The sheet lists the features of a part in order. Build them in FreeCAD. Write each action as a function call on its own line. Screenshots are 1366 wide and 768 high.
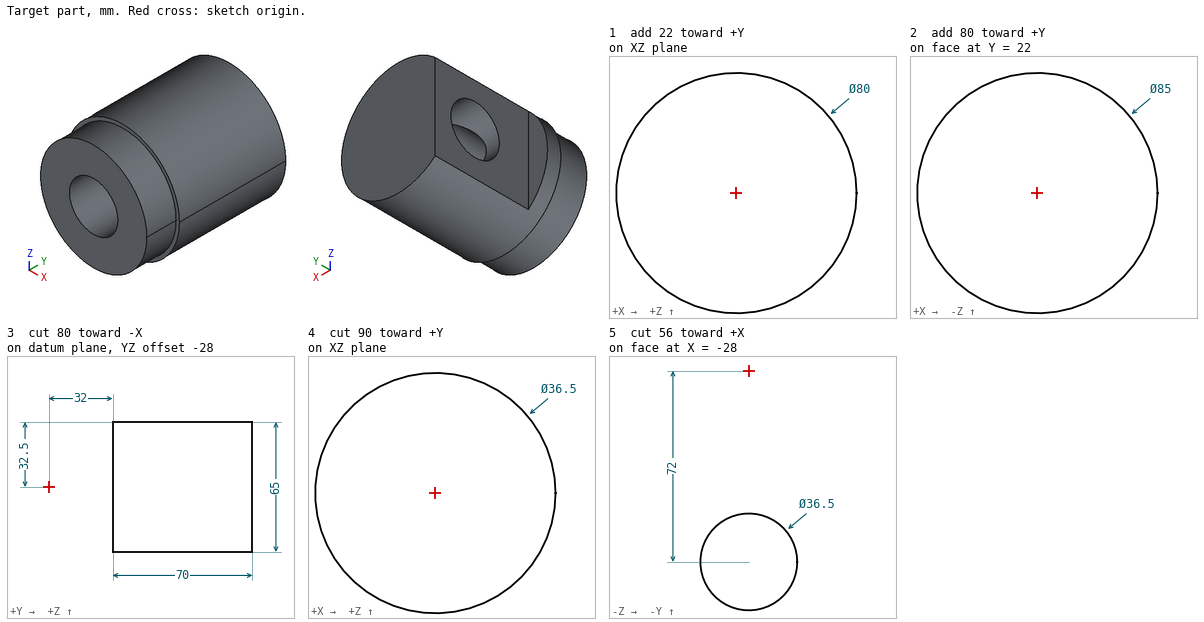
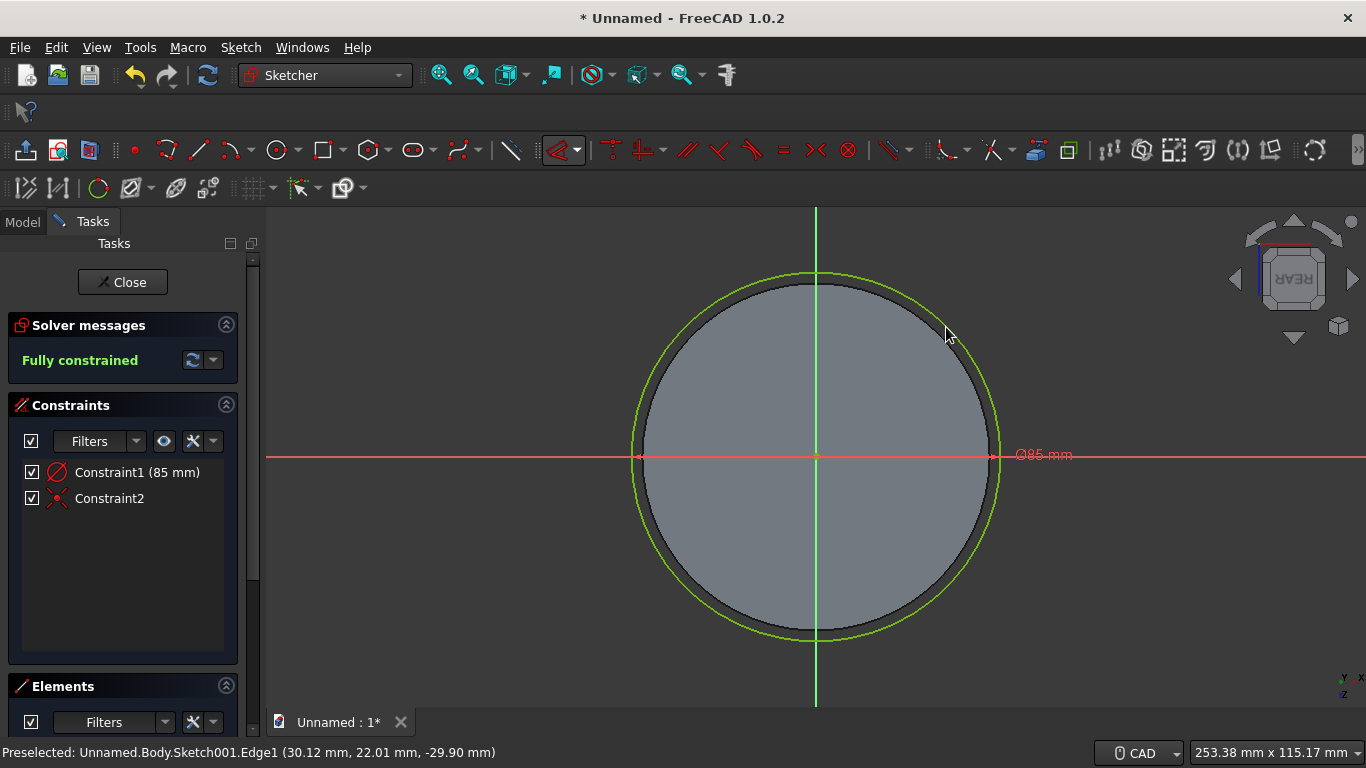
click(123, 282)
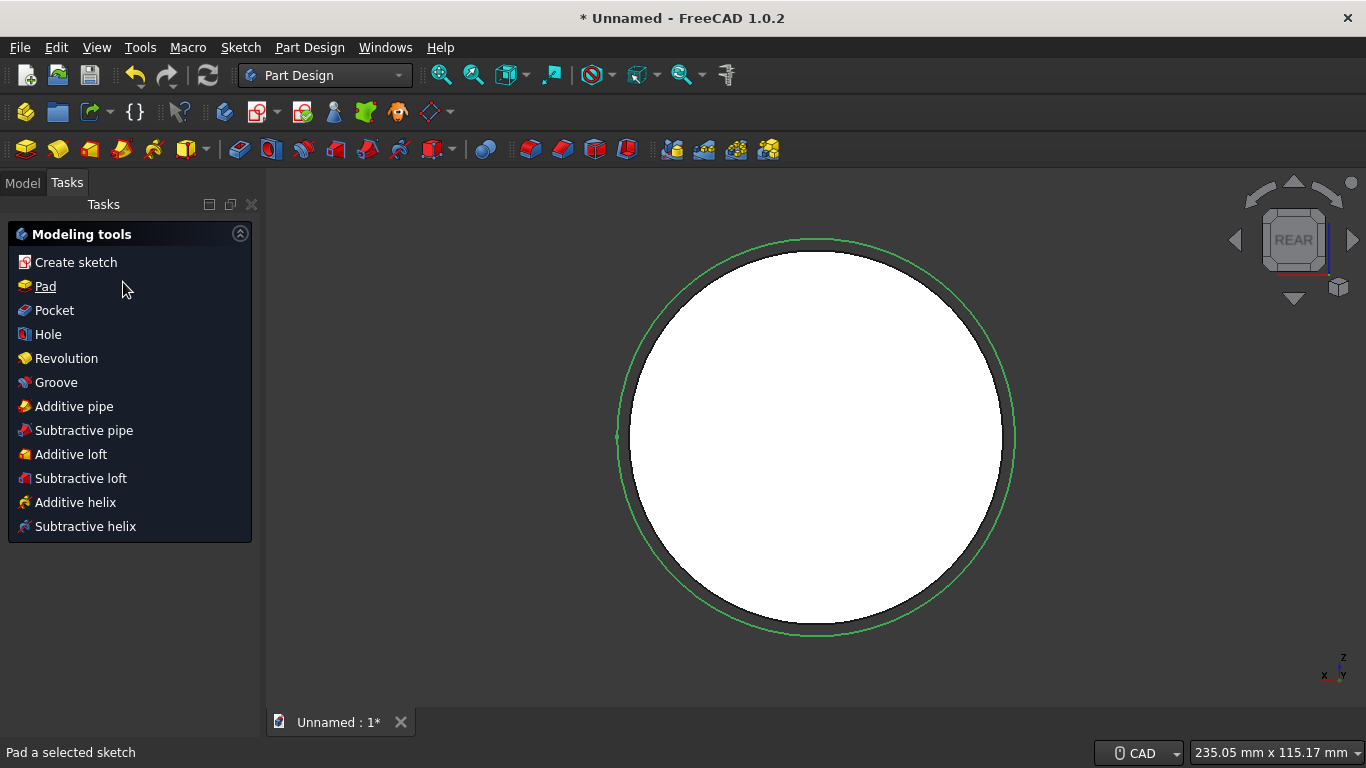
click(26, 150)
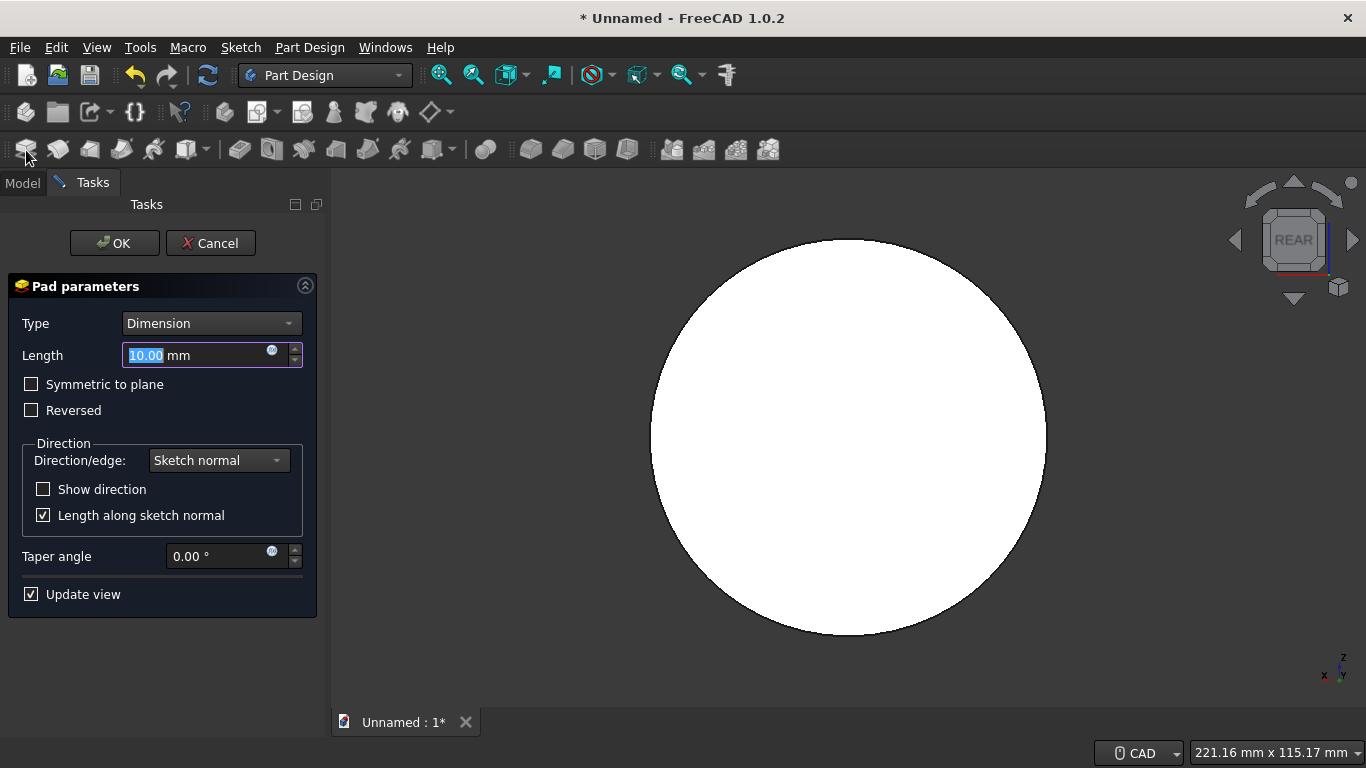
text(80)
key(Tab)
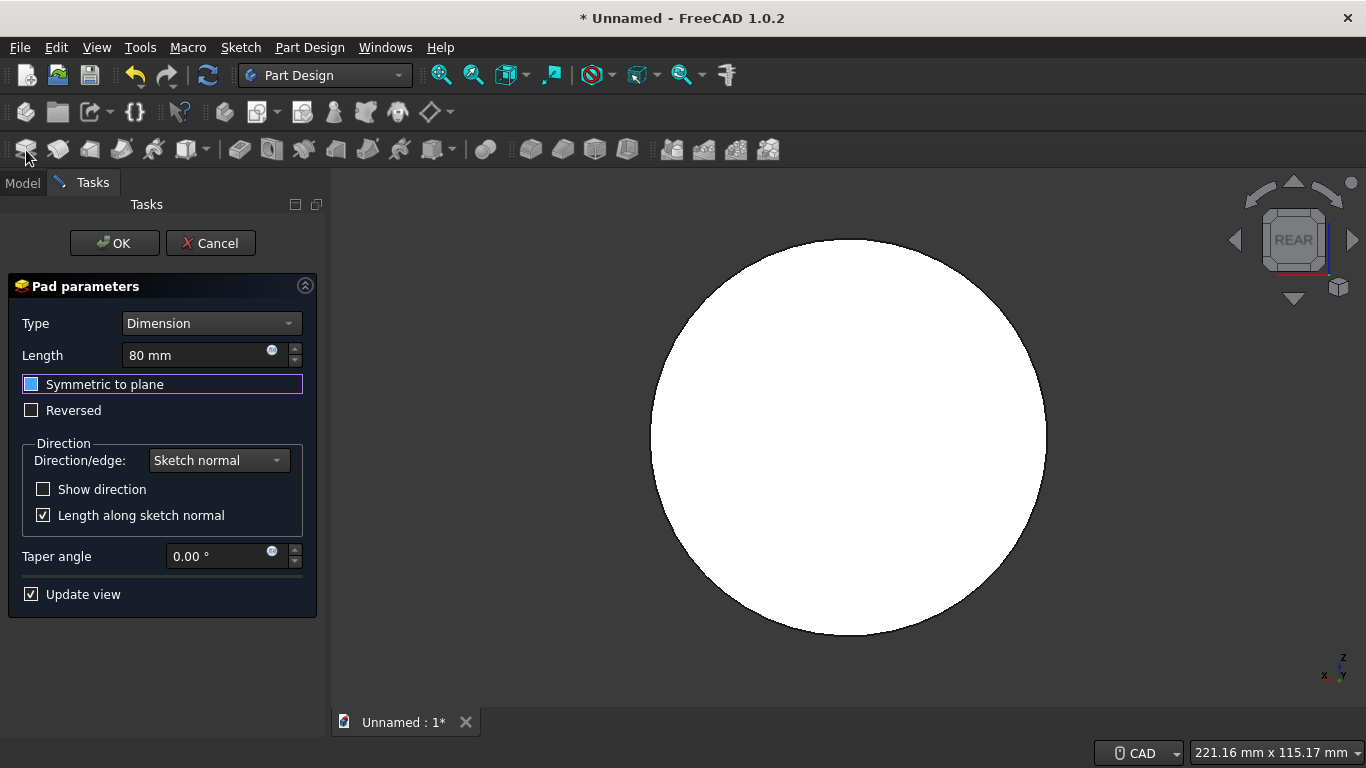
click(115, 243)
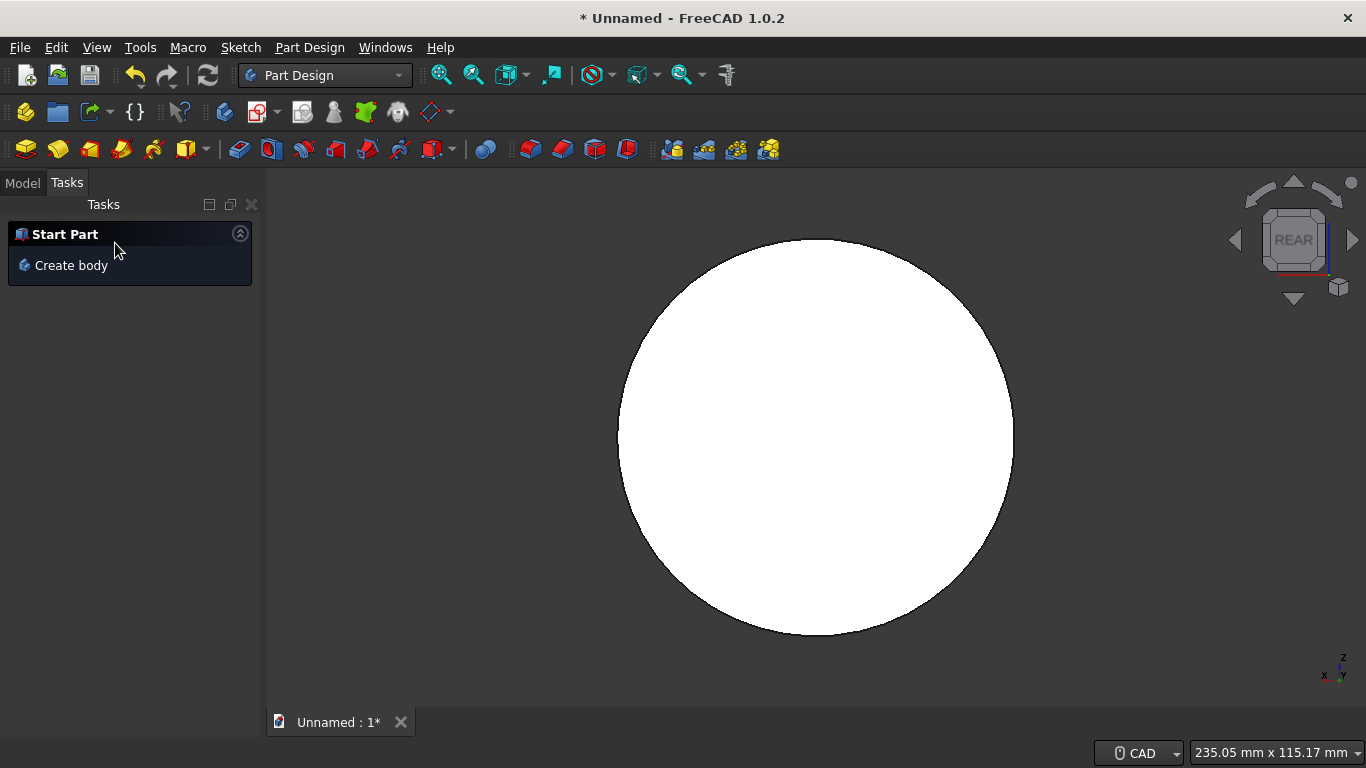
click(23, 182)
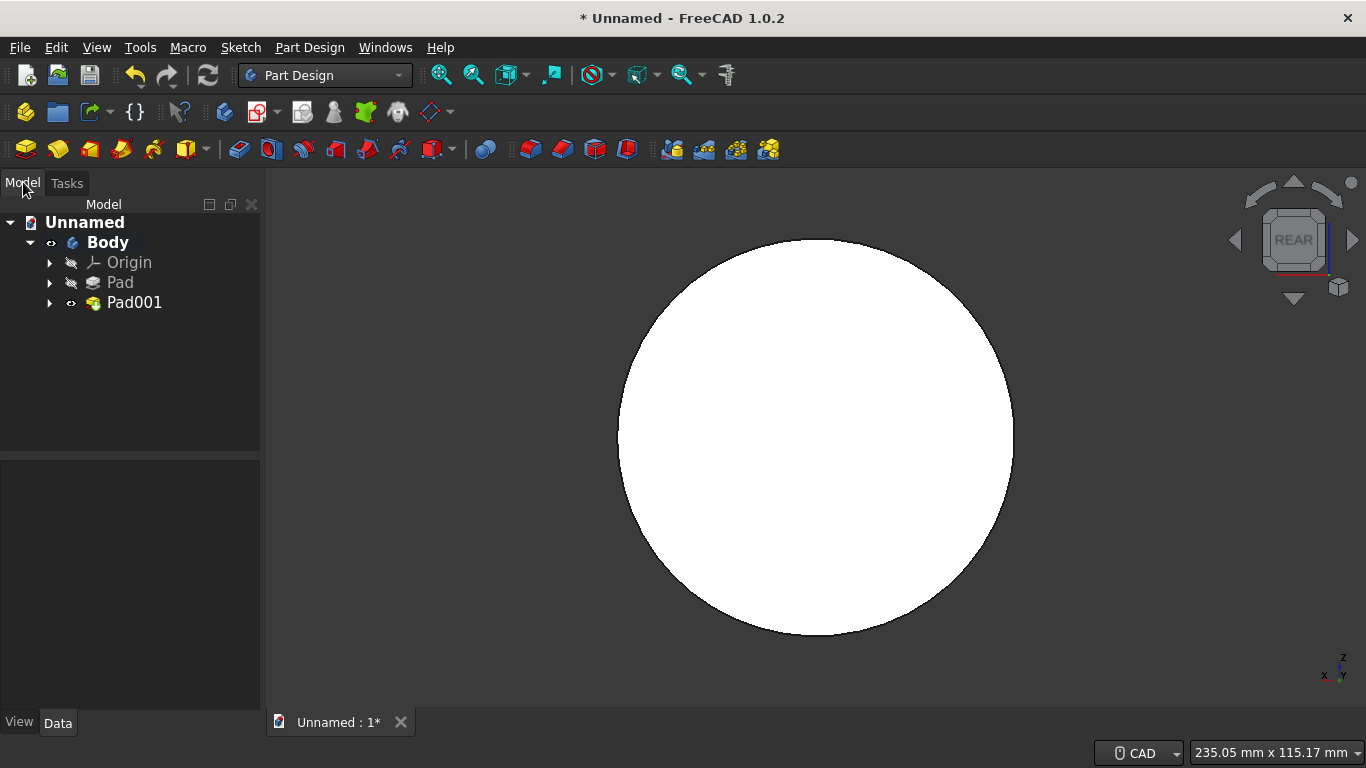
click(50, 263)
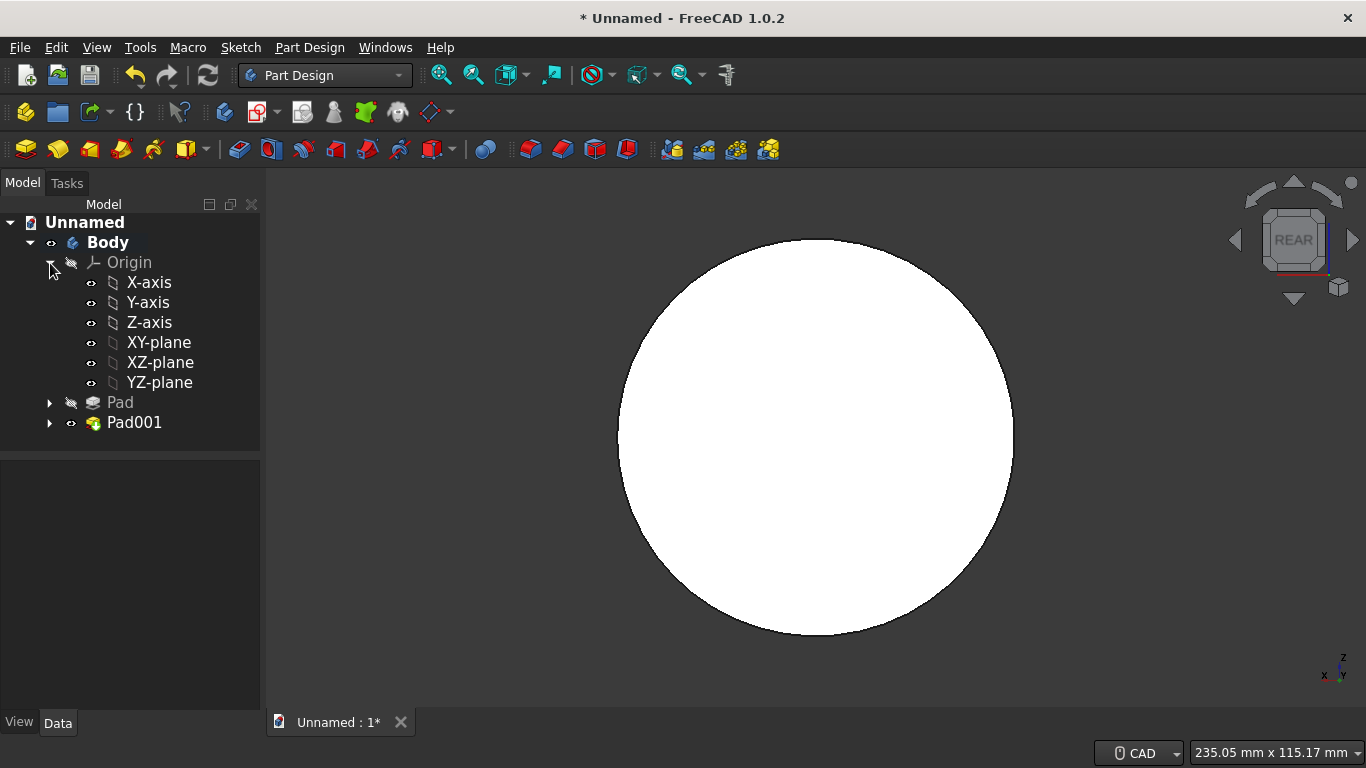
click(136, 383)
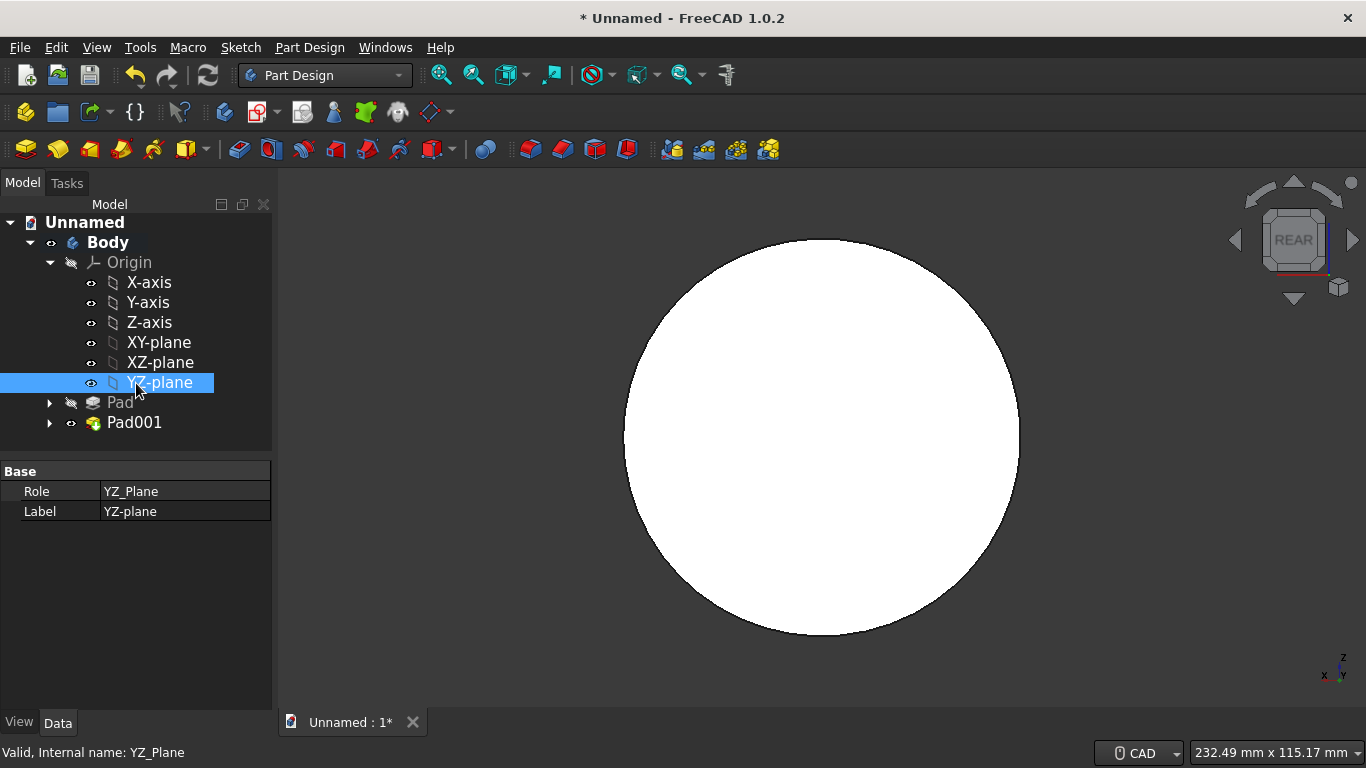
click(430, 112)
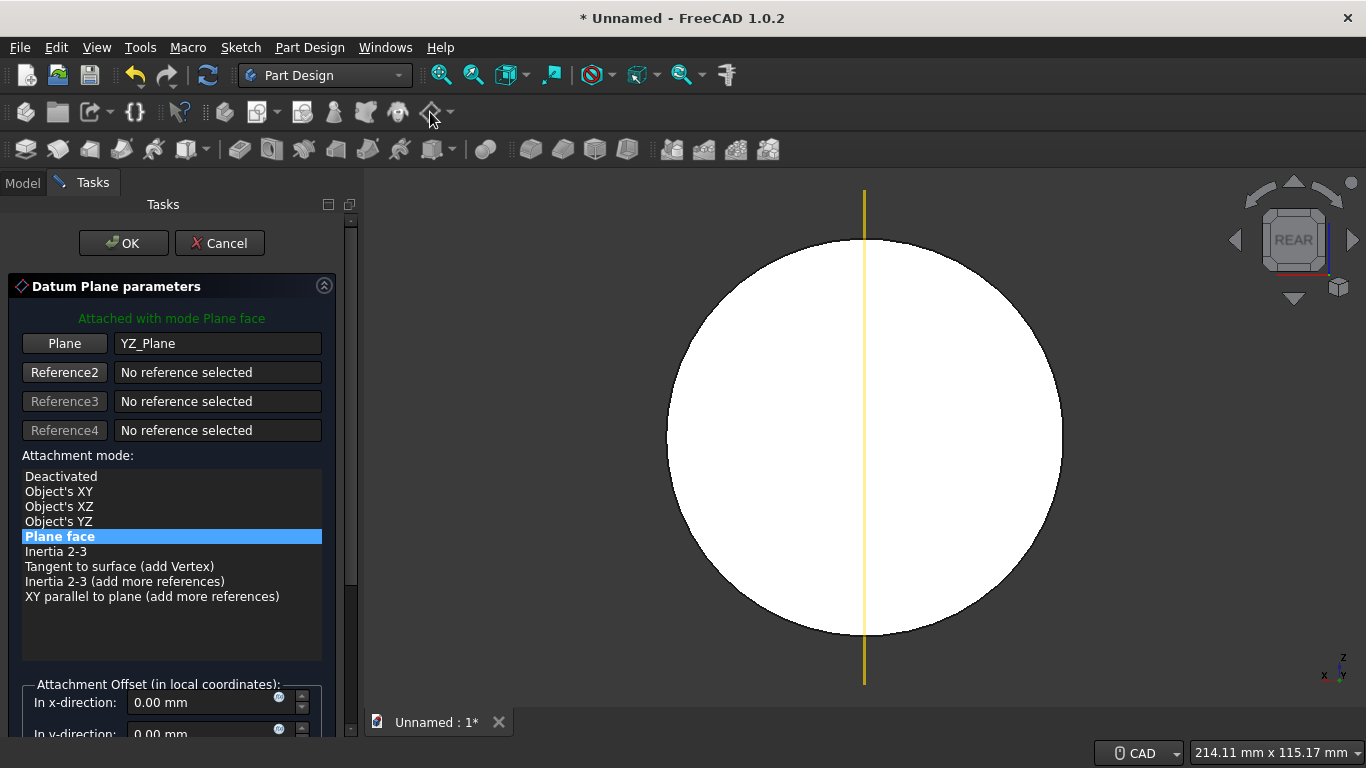
scroll(351, 475, down, 2)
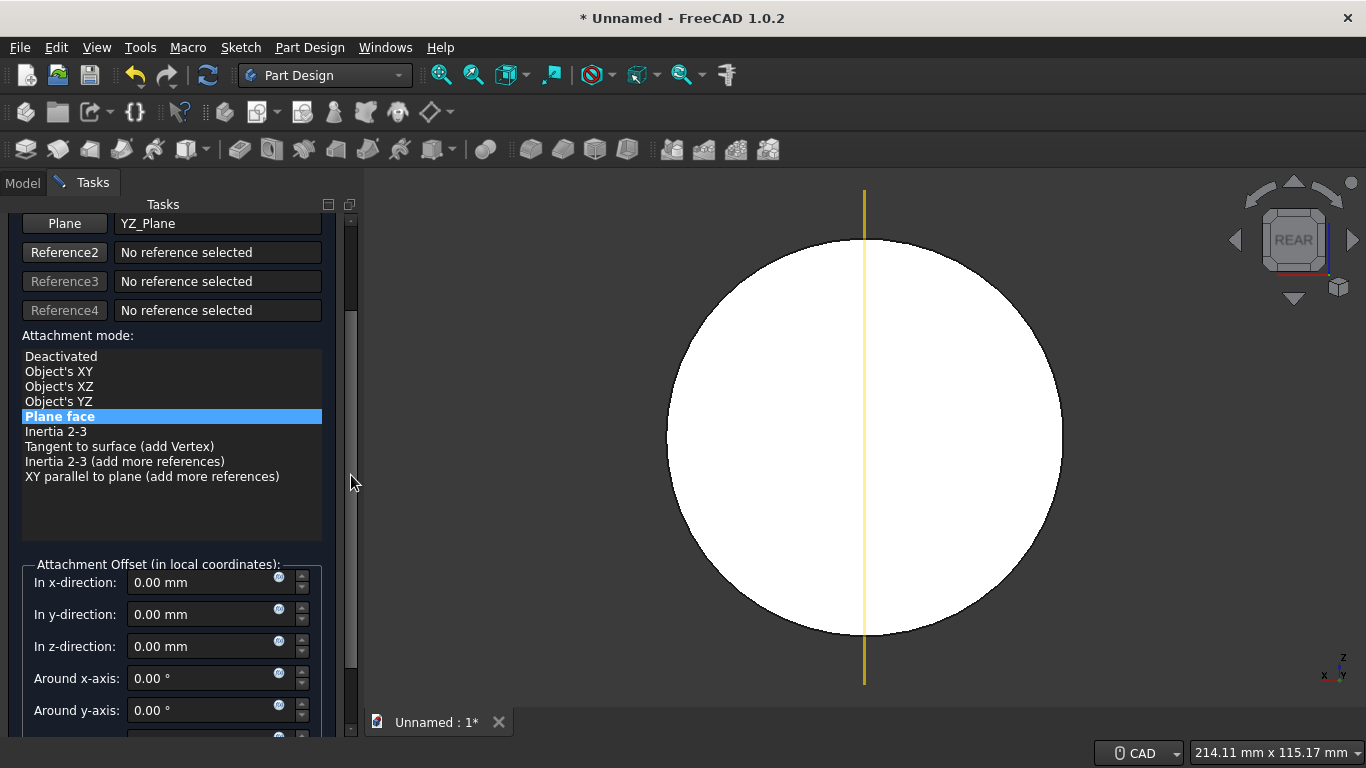
triple_click(210, 646)